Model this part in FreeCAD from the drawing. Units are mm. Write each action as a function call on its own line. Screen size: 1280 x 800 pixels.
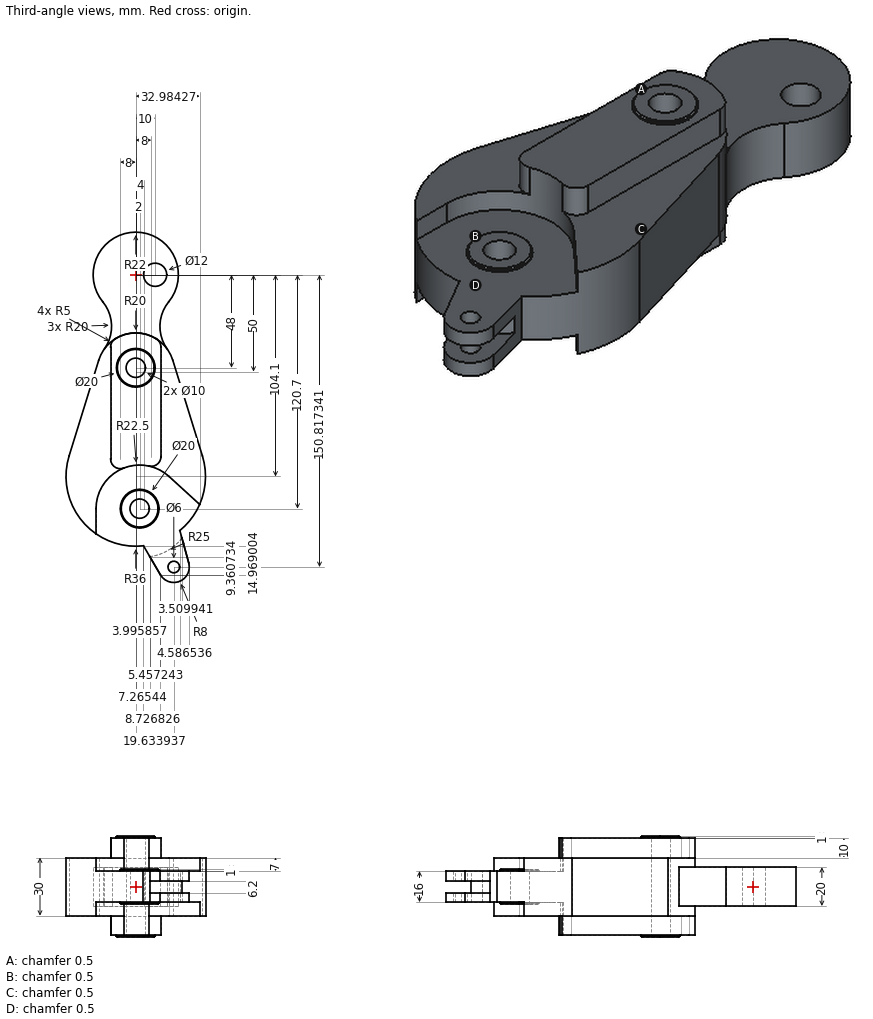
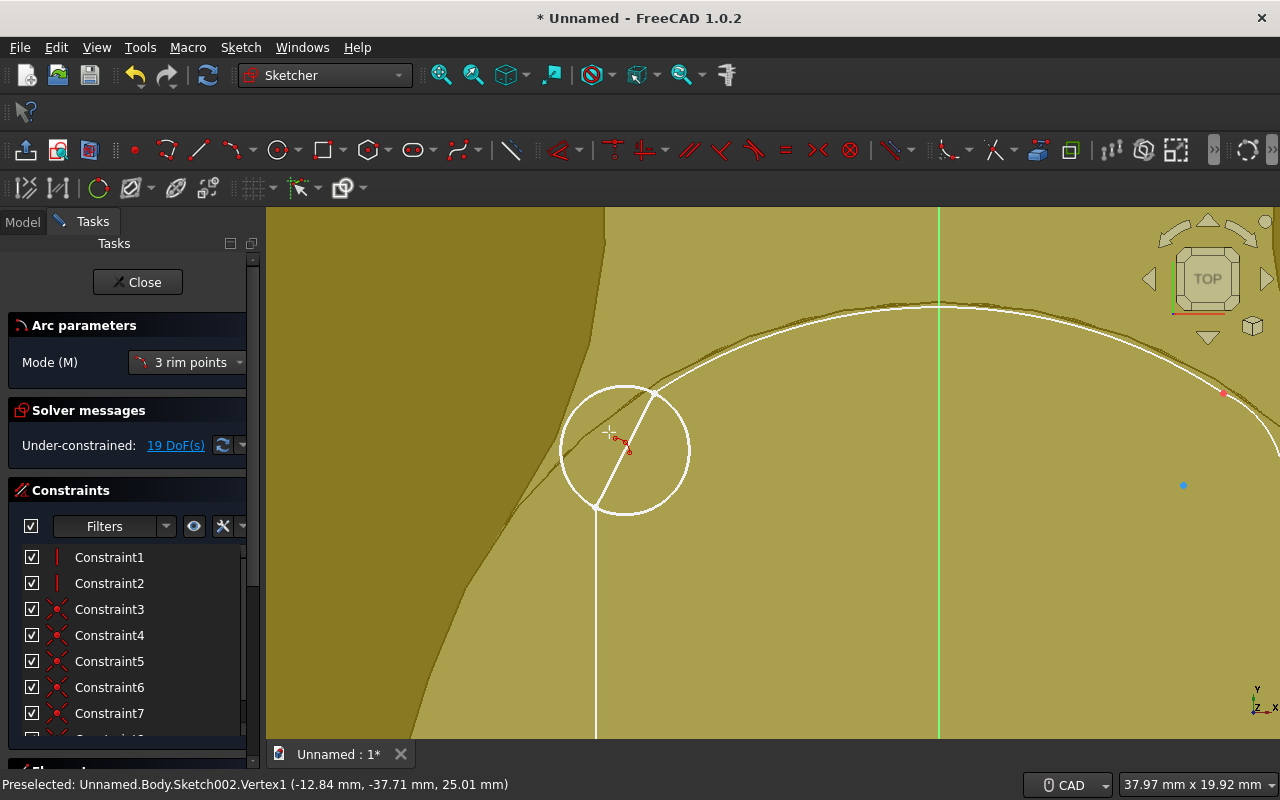
click(608, 433)
key(Escape)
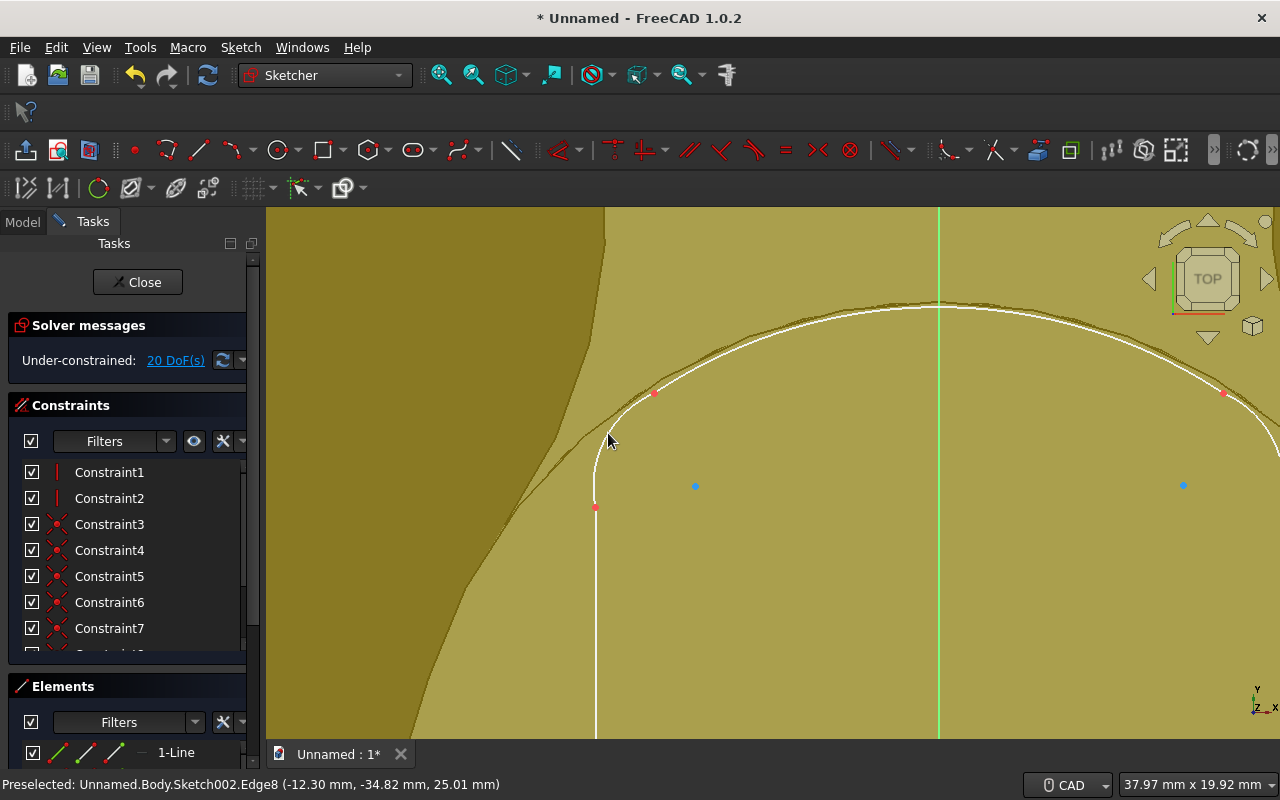
scroll(668, 417, down, 10)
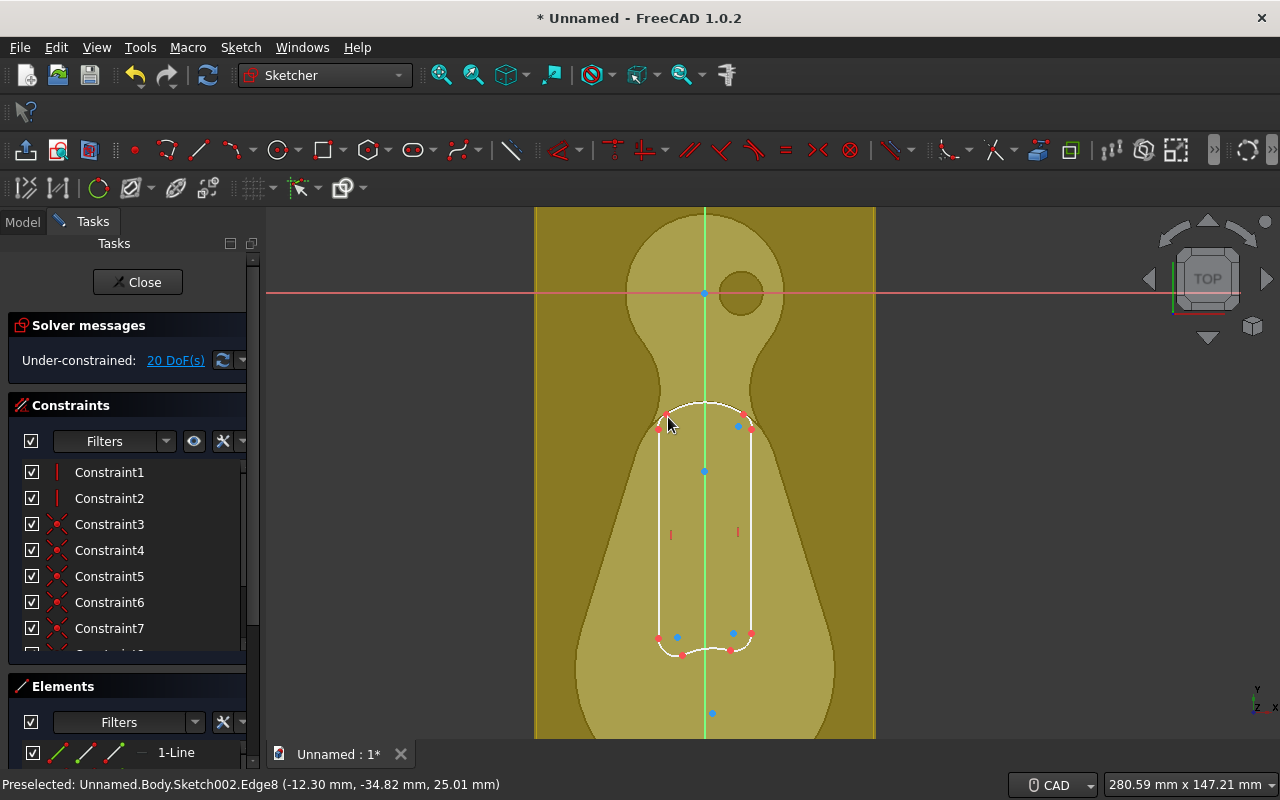
click(659, 492)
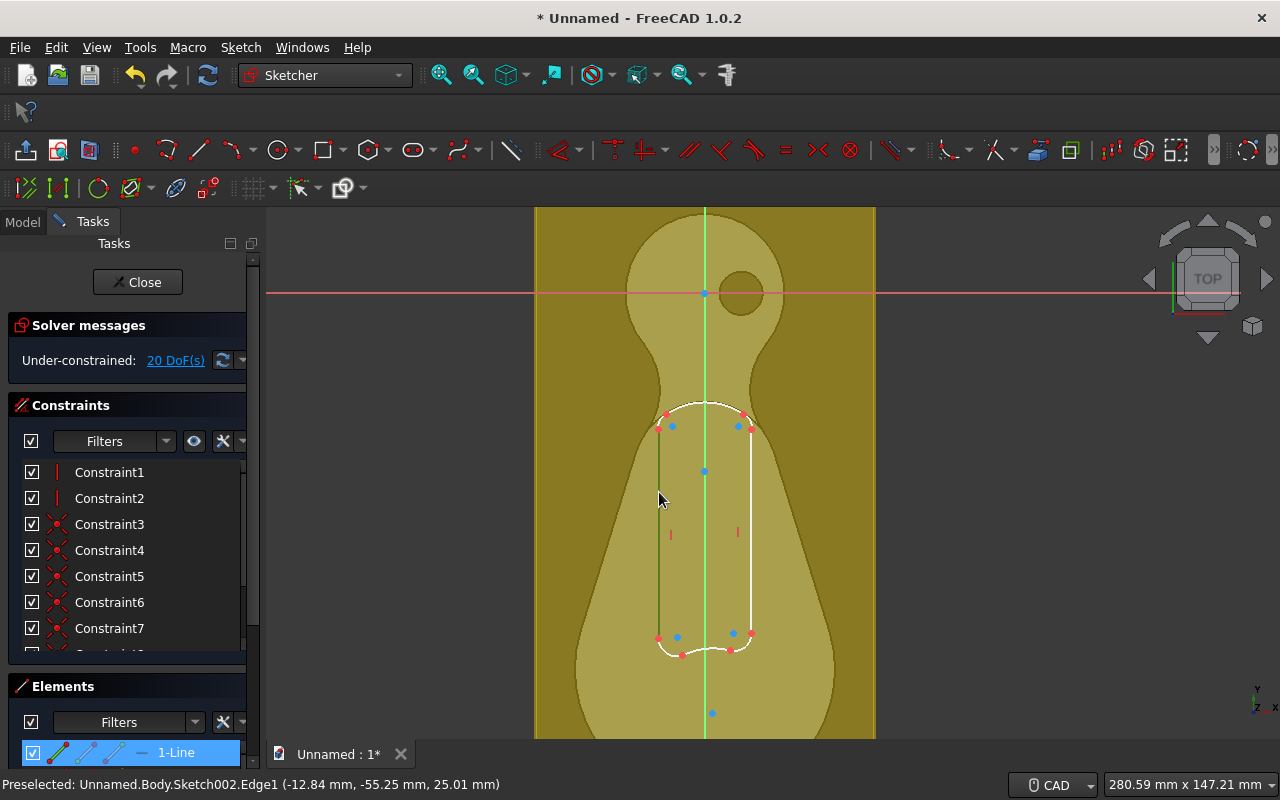
scroll(662, 648, up, 2)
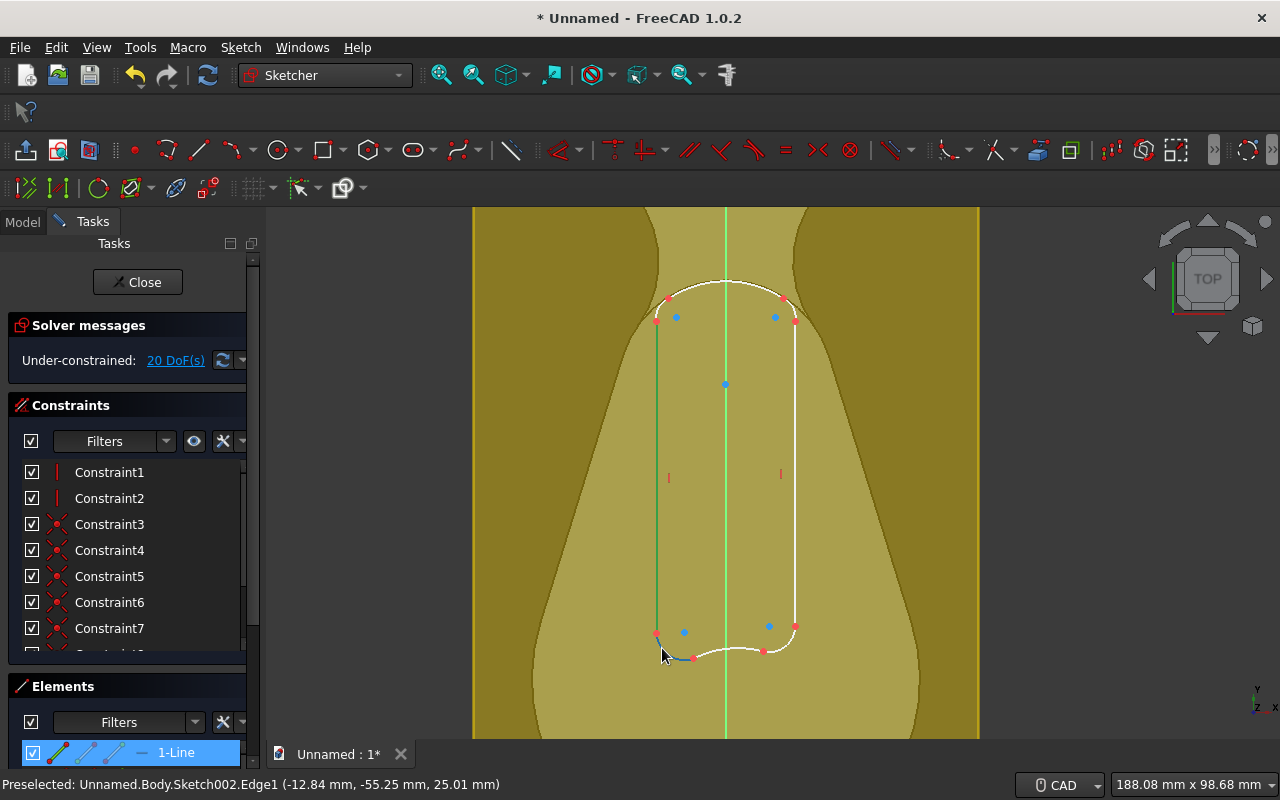
click(661, 648)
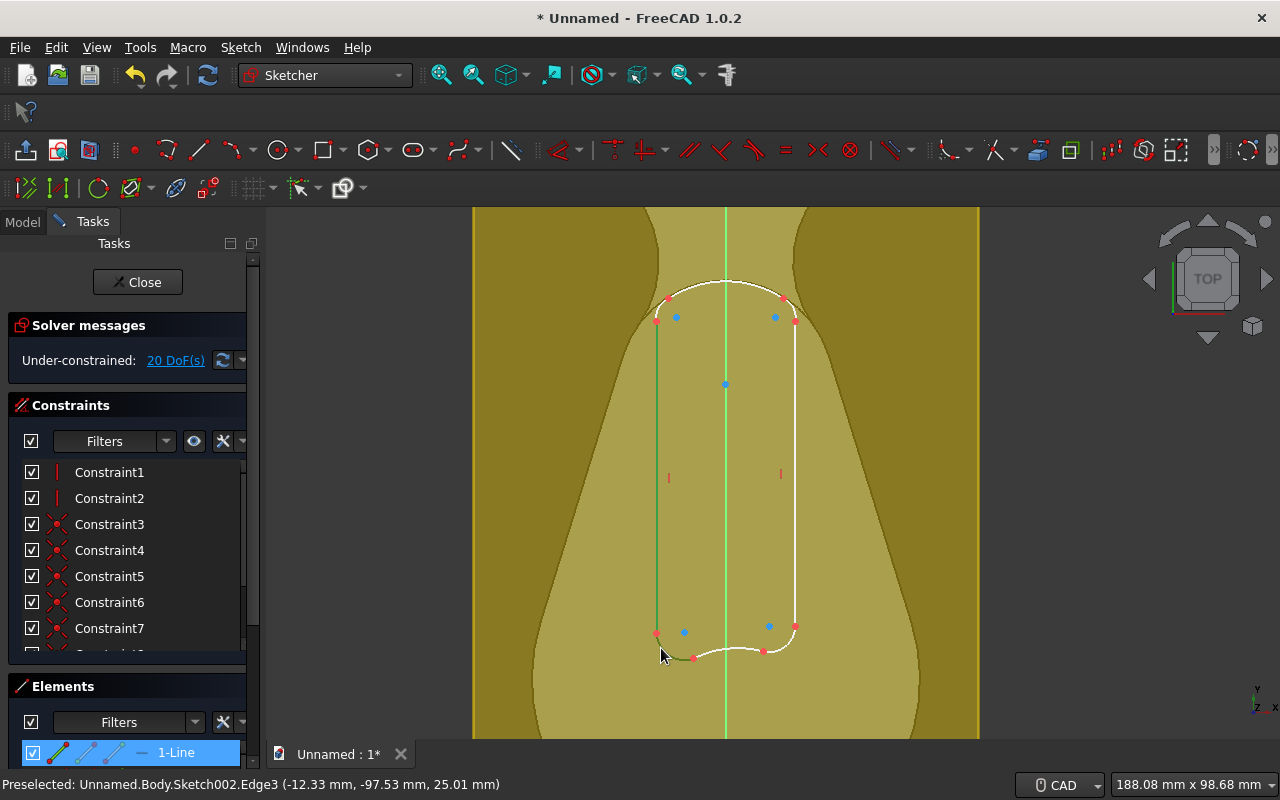
click(754, 150)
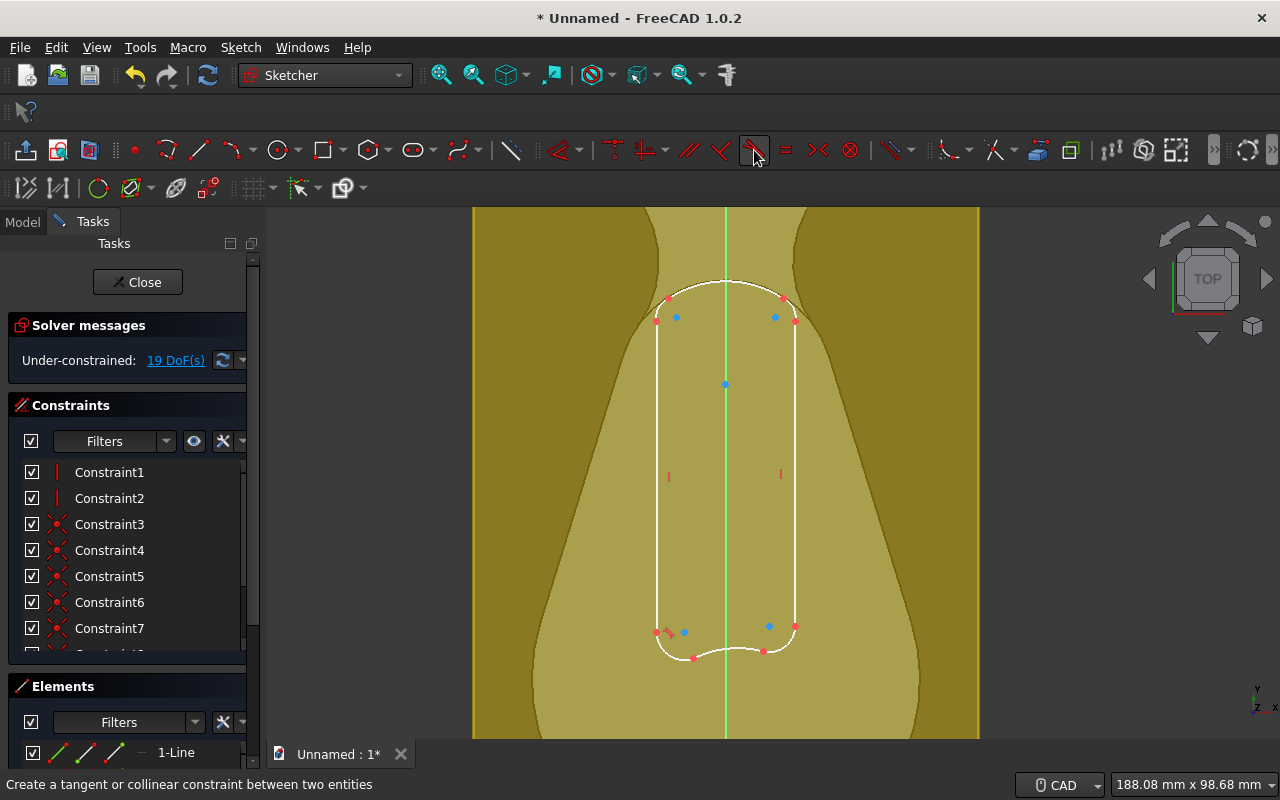
click(657, 415)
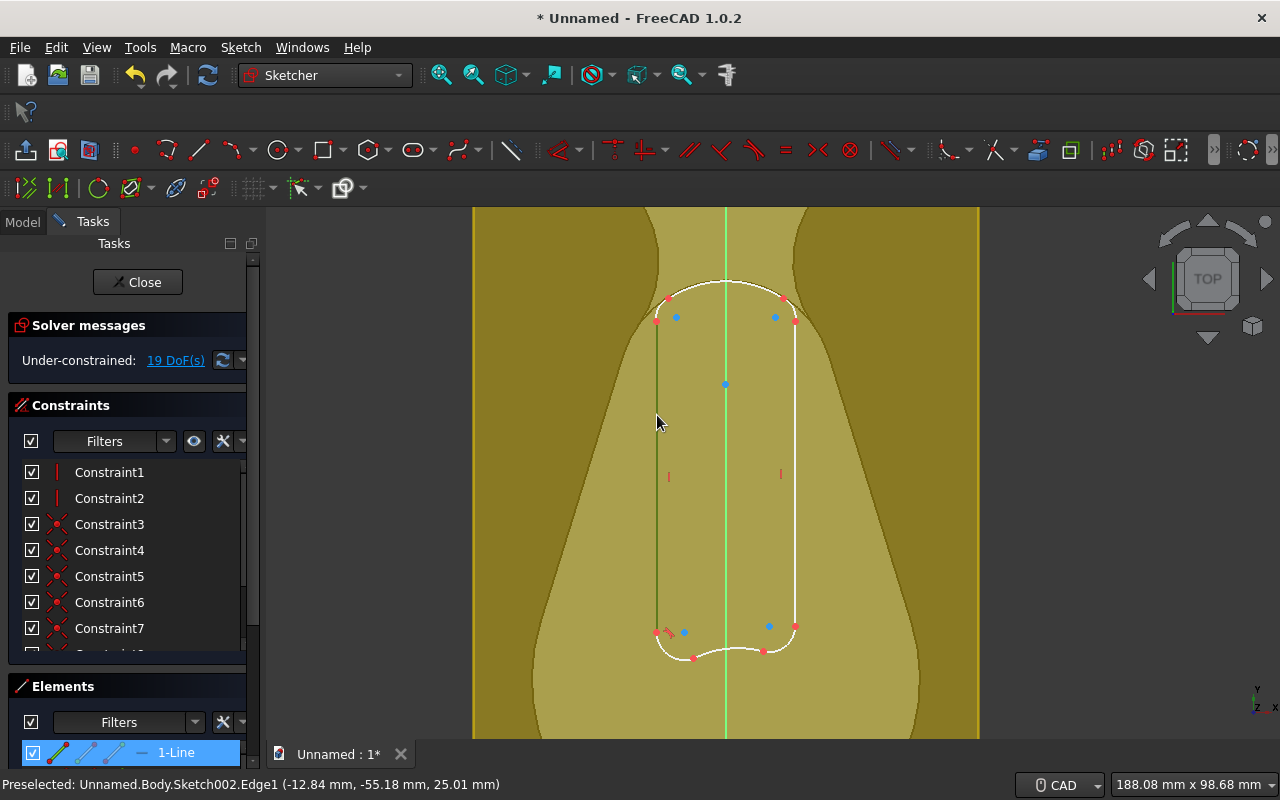
click(658, 308)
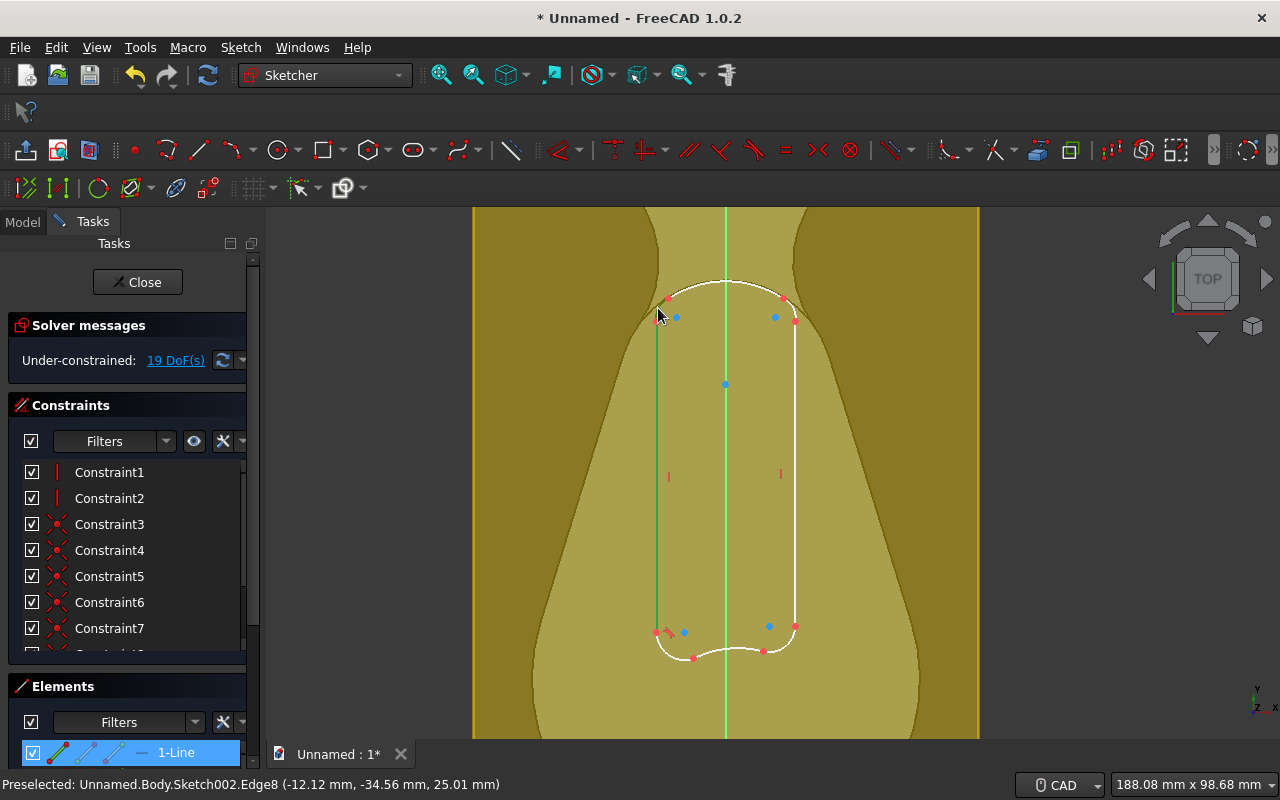
click(754, 150)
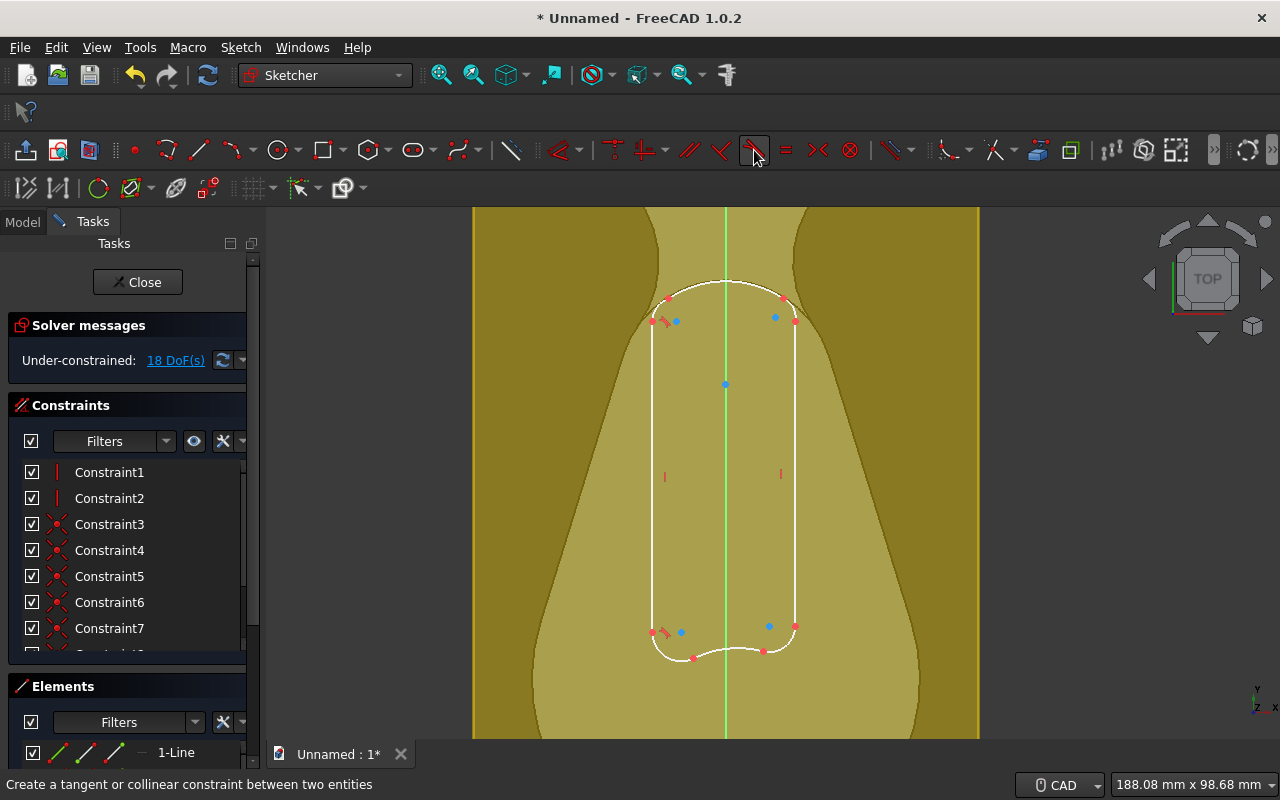
click(795, 535)